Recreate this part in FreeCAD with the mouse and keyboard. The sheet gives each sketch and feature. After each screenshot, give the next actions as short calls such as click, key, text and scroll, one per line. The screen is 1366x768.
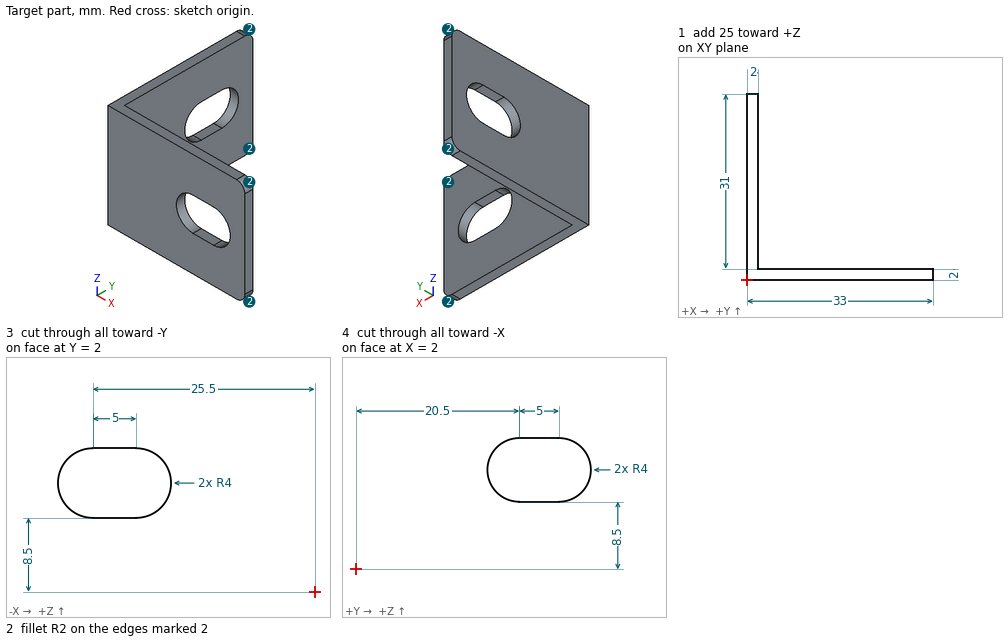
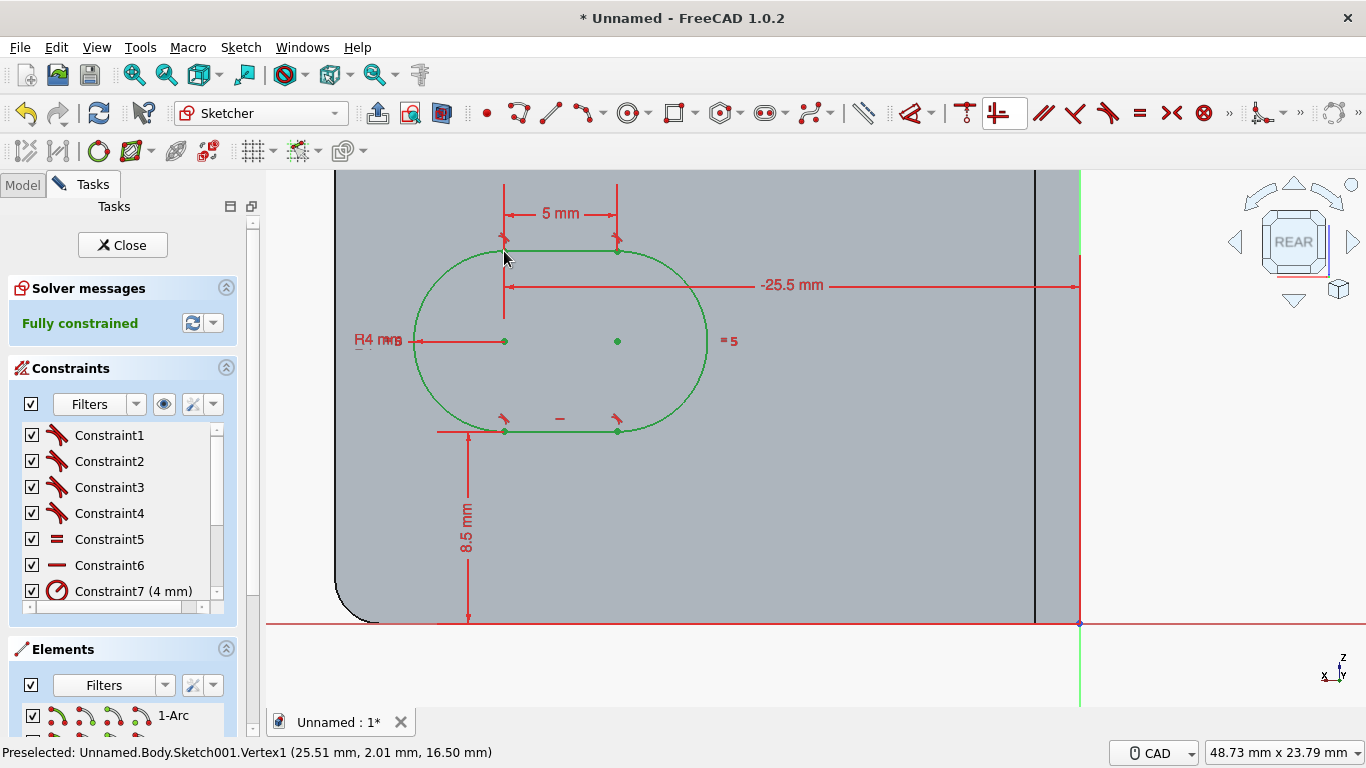
click(123, 245)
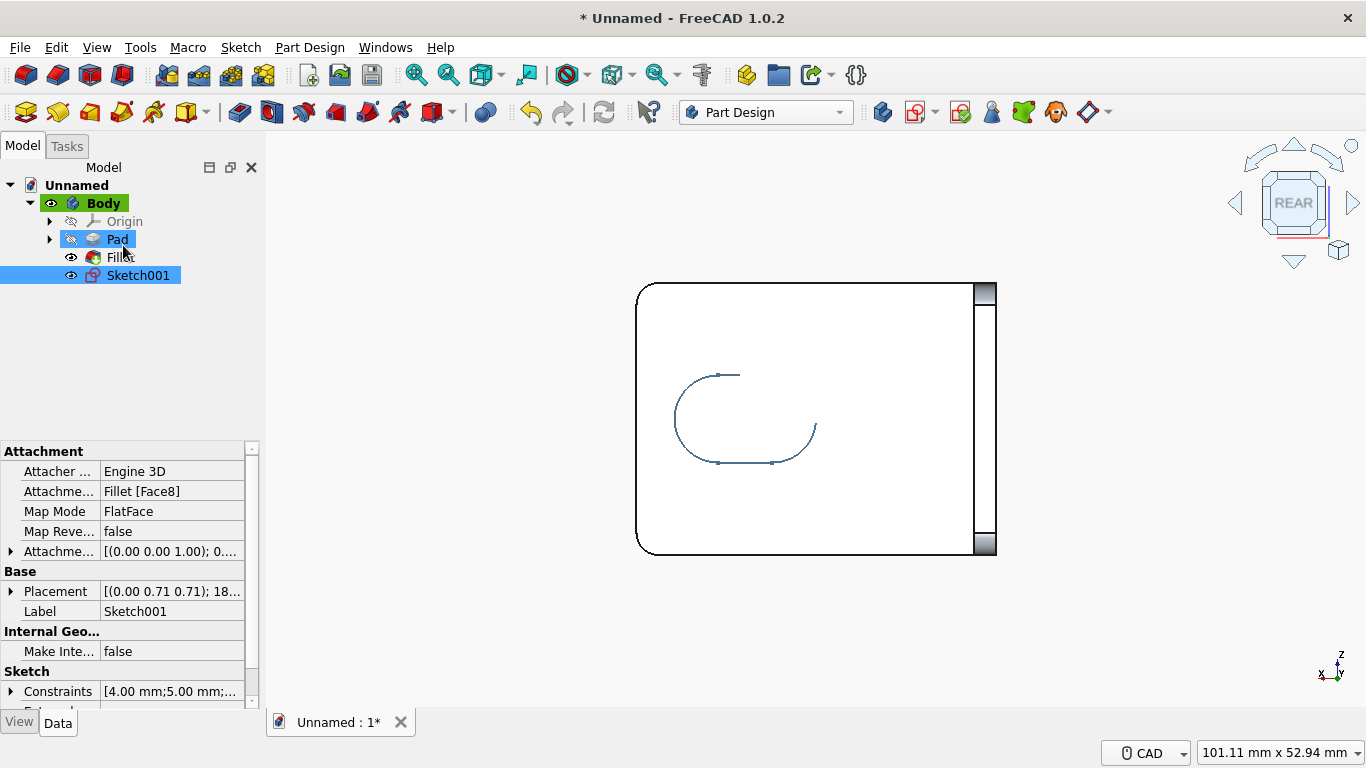
click(240, 112)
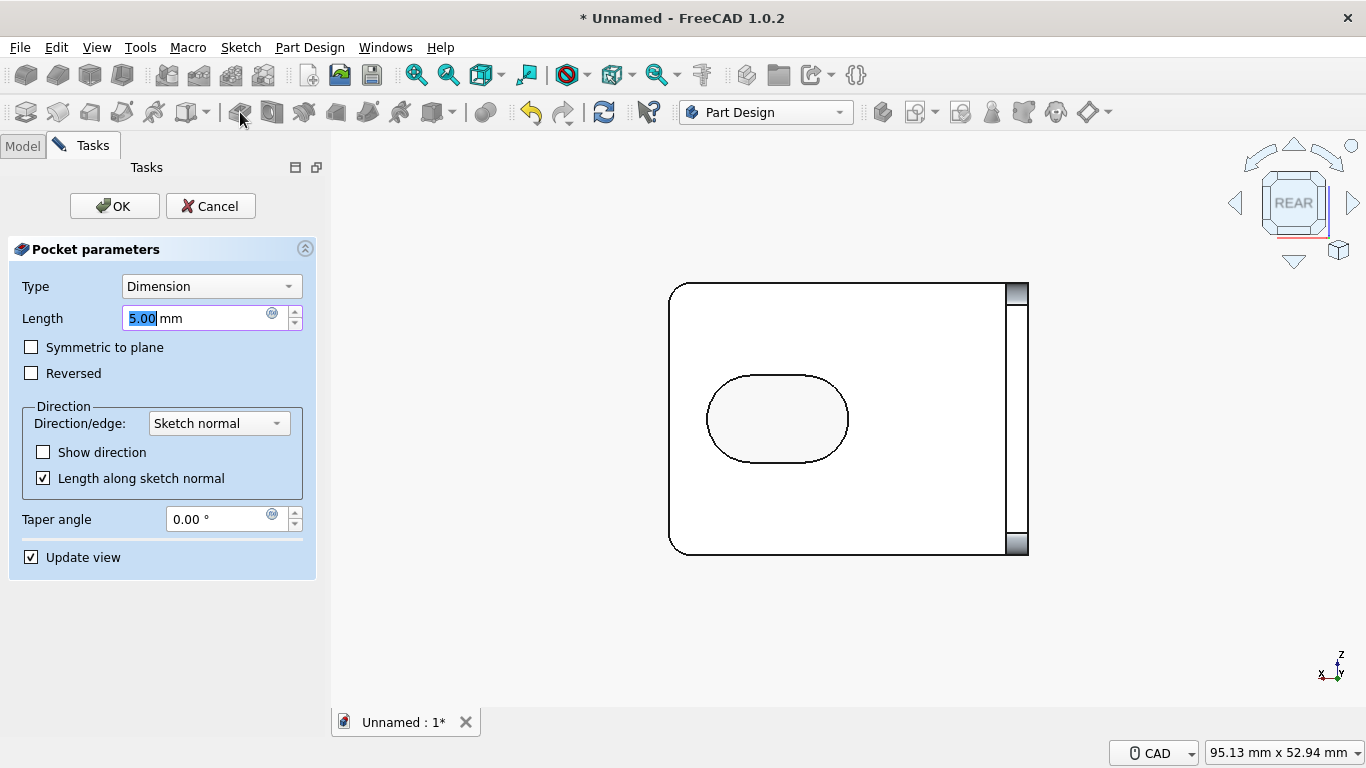
click(212, 286)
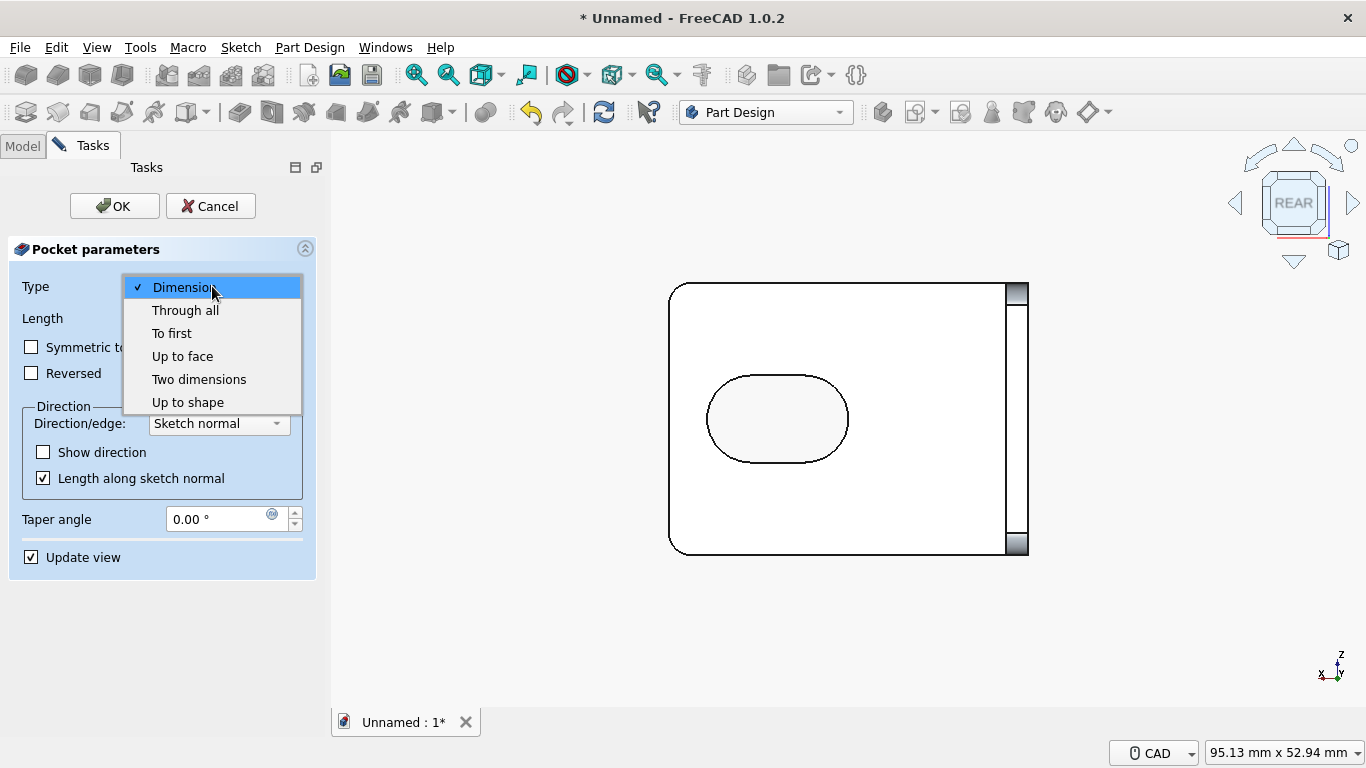
click(212, 310)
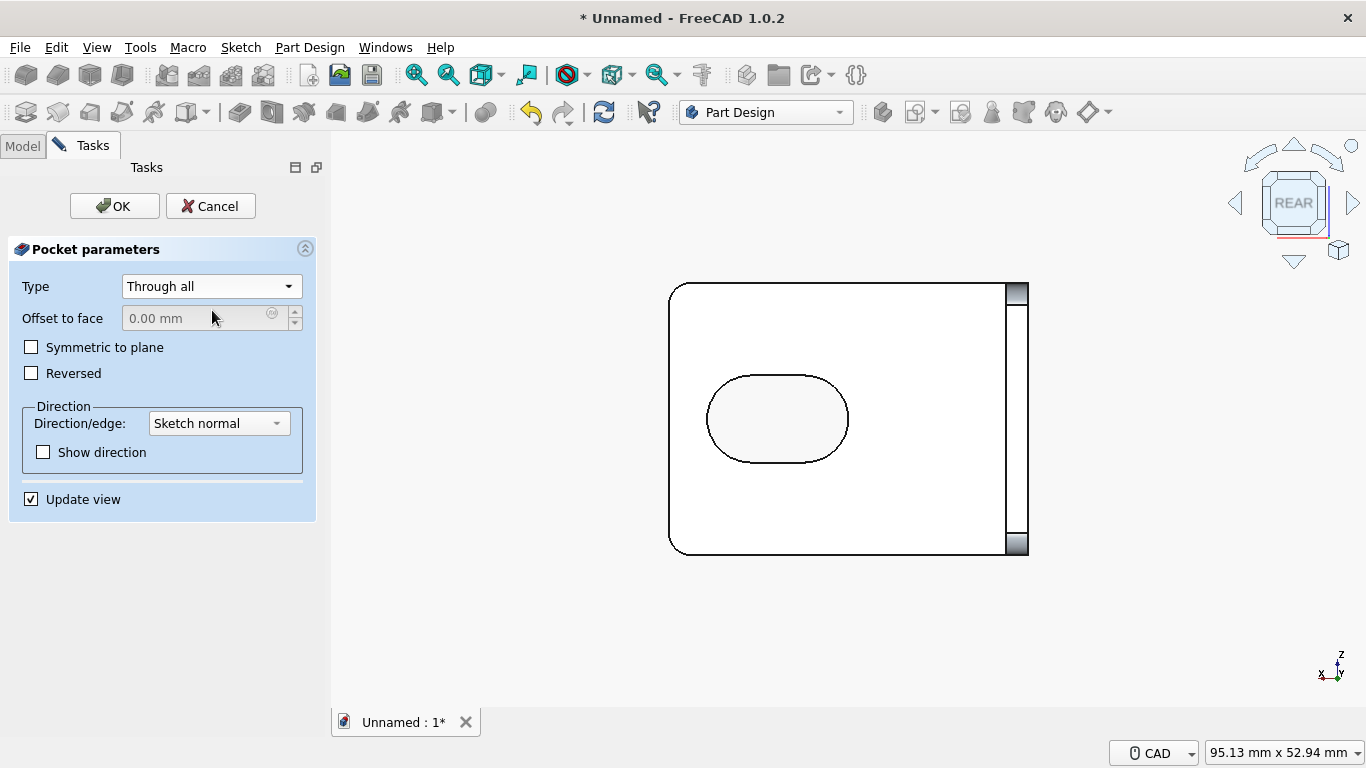
click(115, 206)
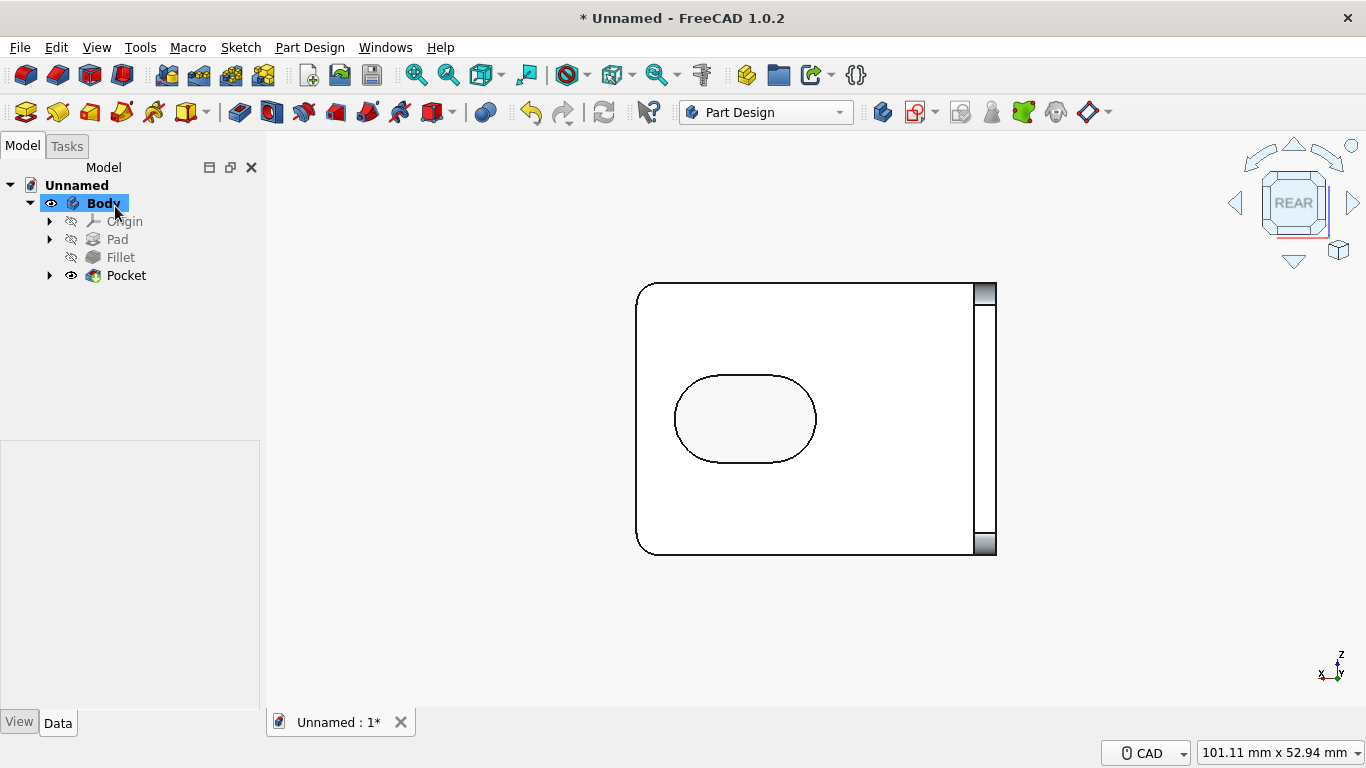
key(0)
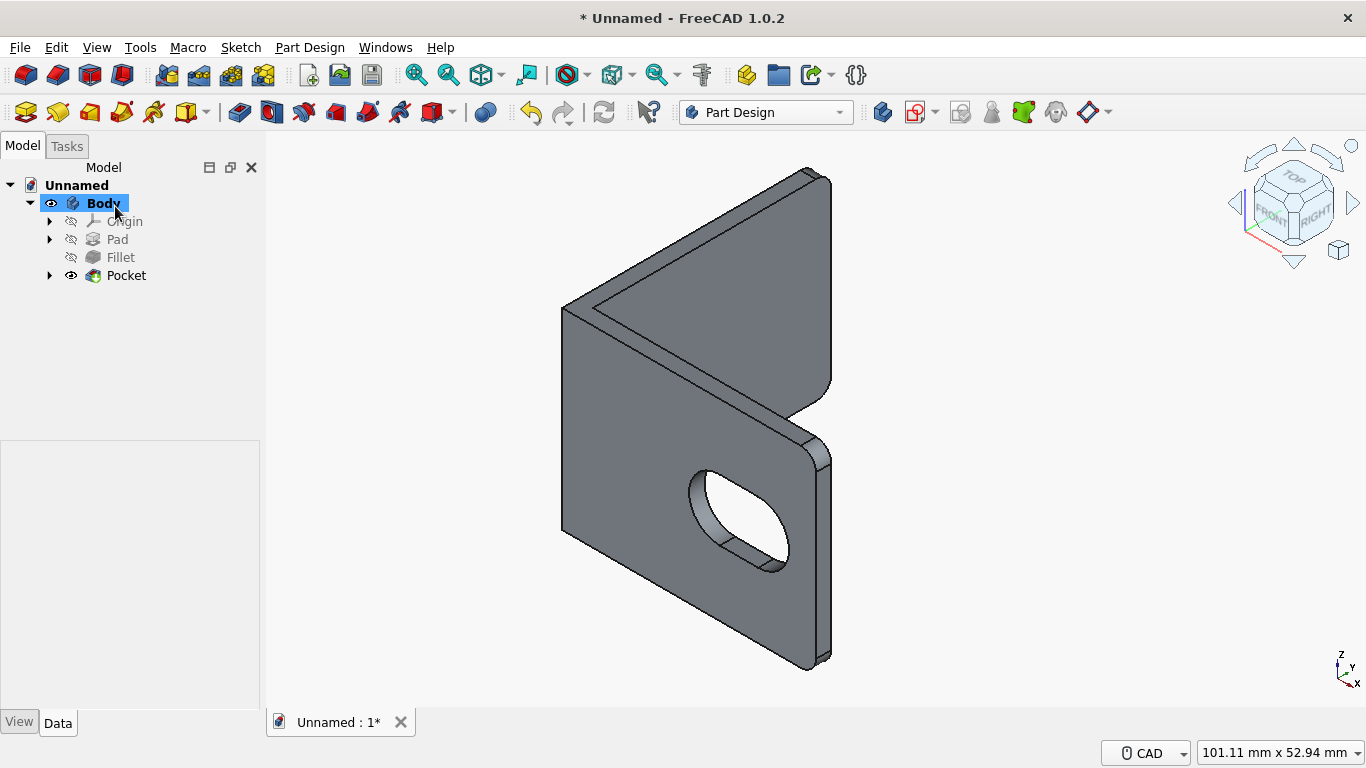
click(712, 349)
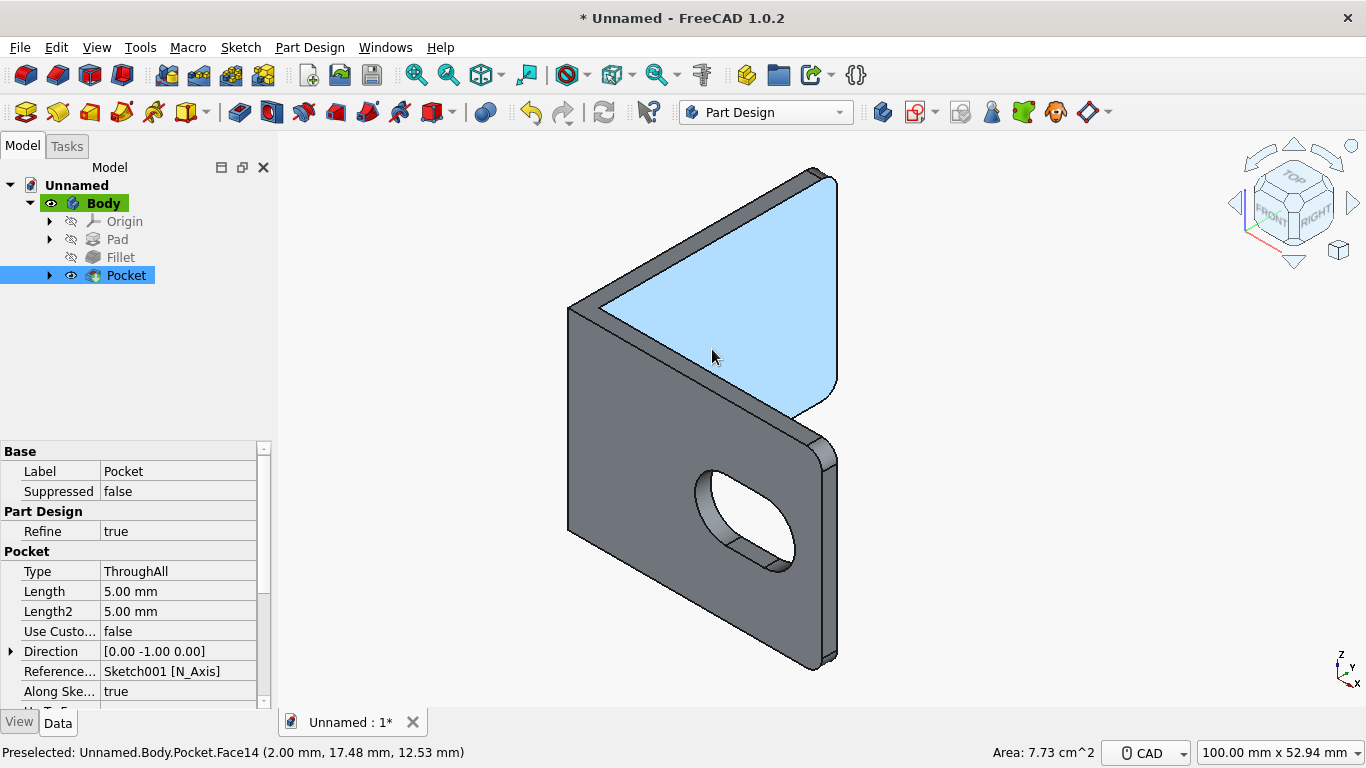
click(916, 112)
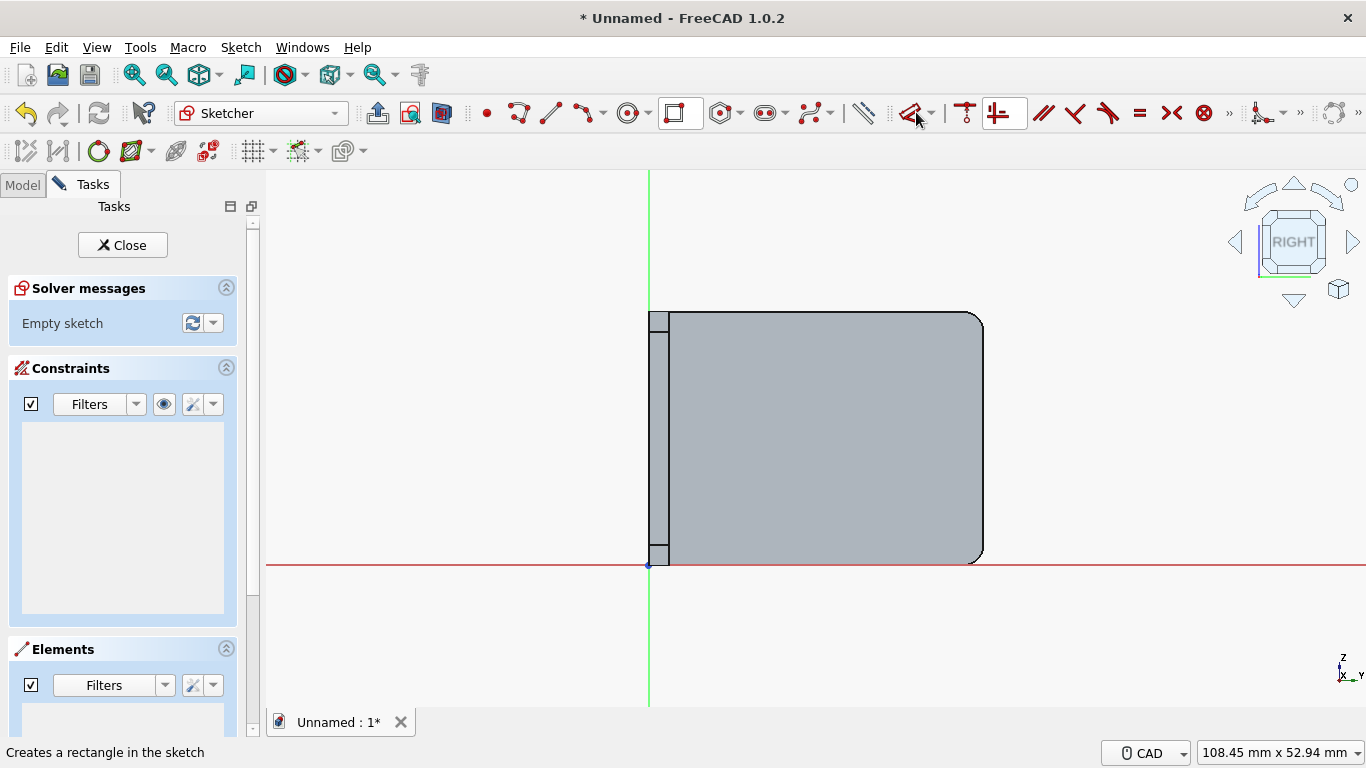
scroll(840, 517, up, 4)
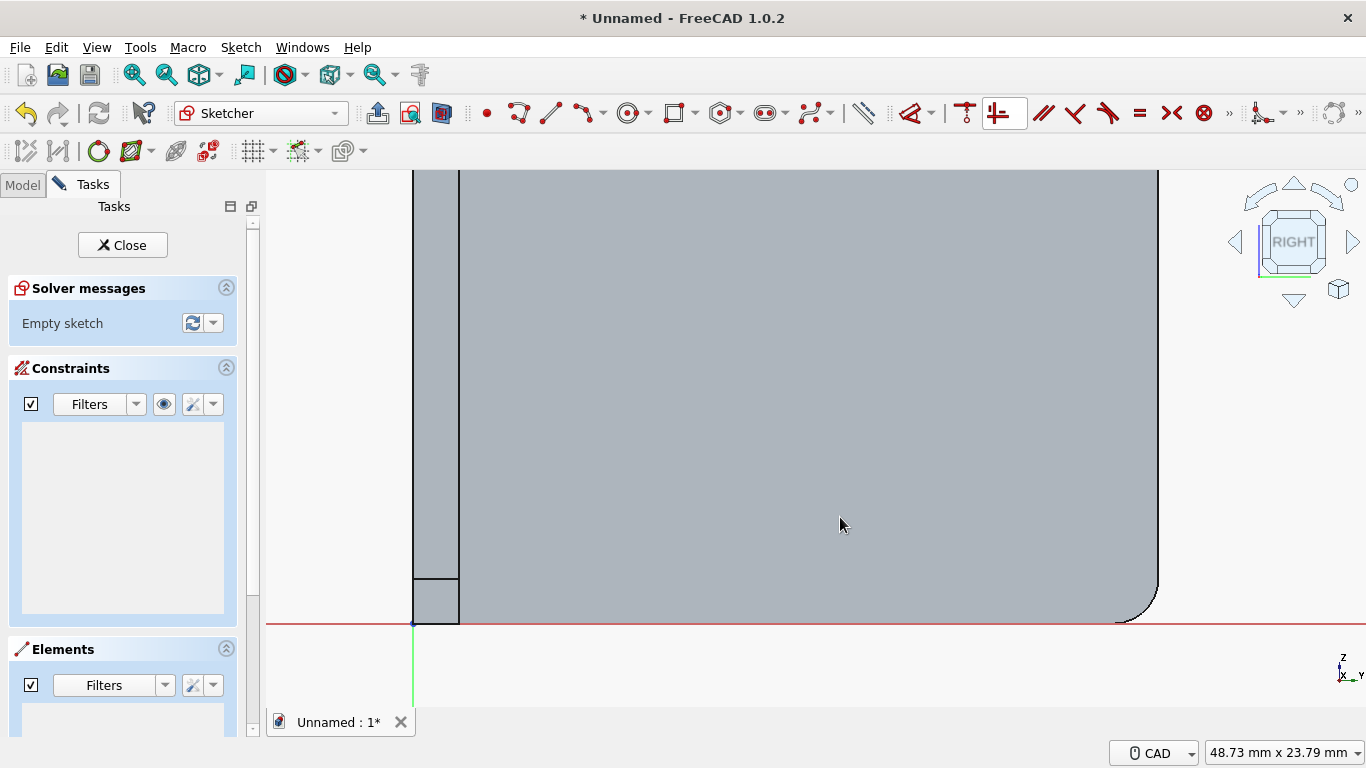
key(g)
key(s)